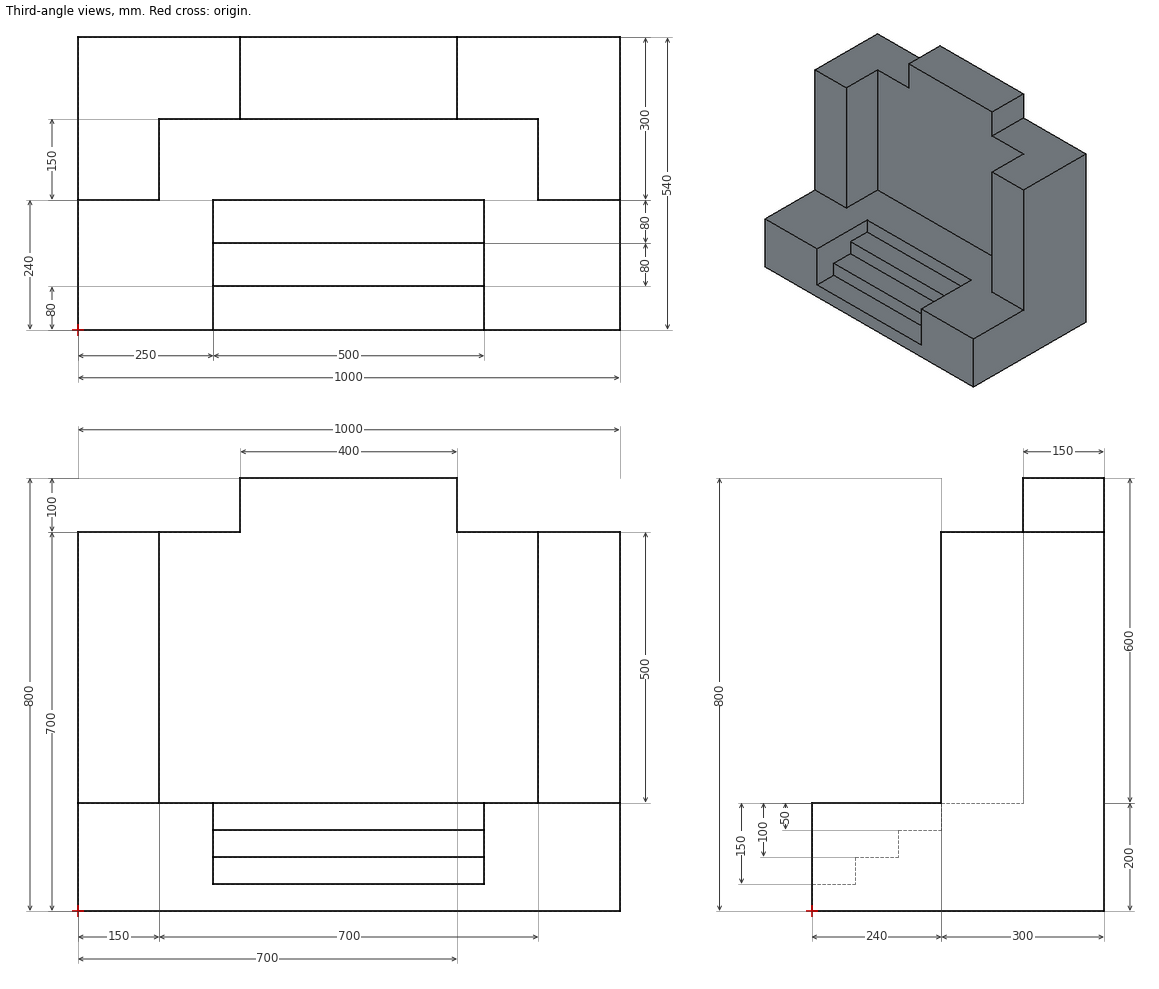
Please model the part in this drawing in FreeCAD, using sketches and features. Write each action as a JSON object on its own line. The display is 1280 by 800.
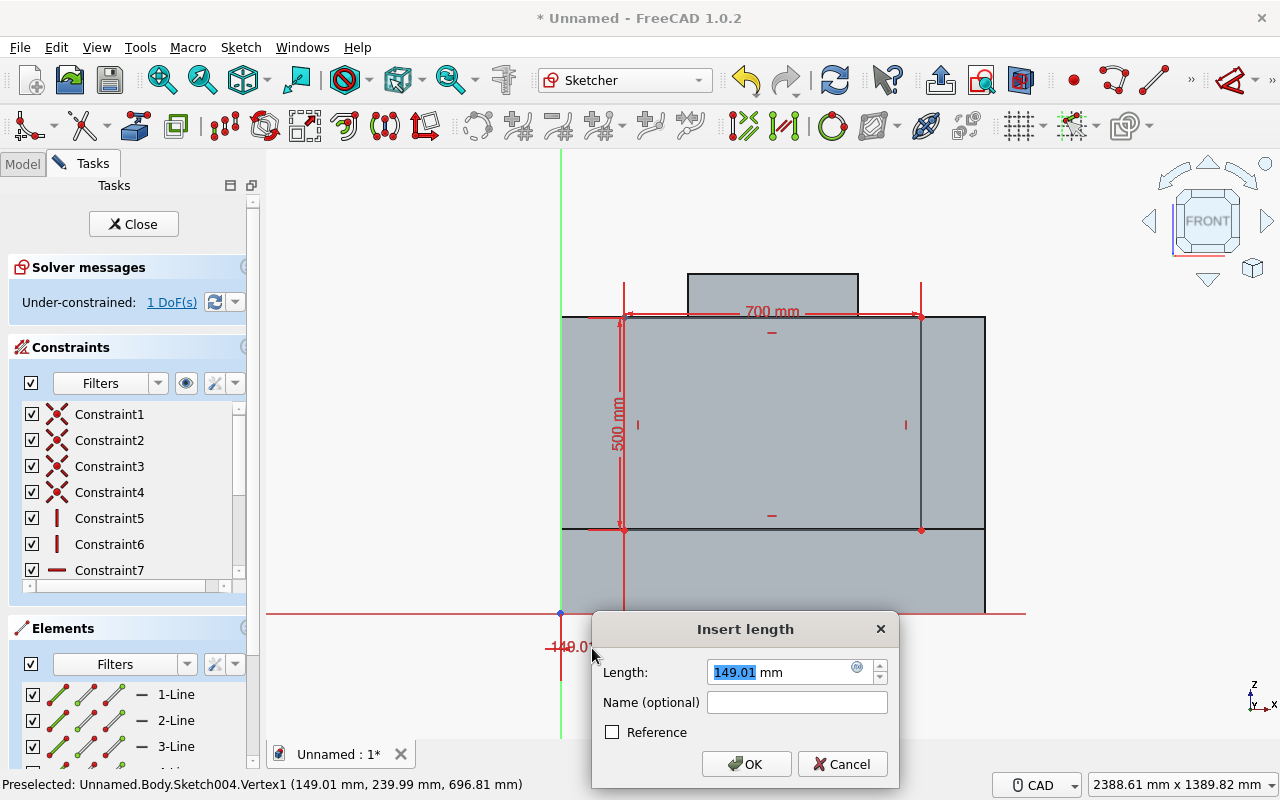
{"action": "type", "text": "150"}
{"action": "key", "text": "Return"}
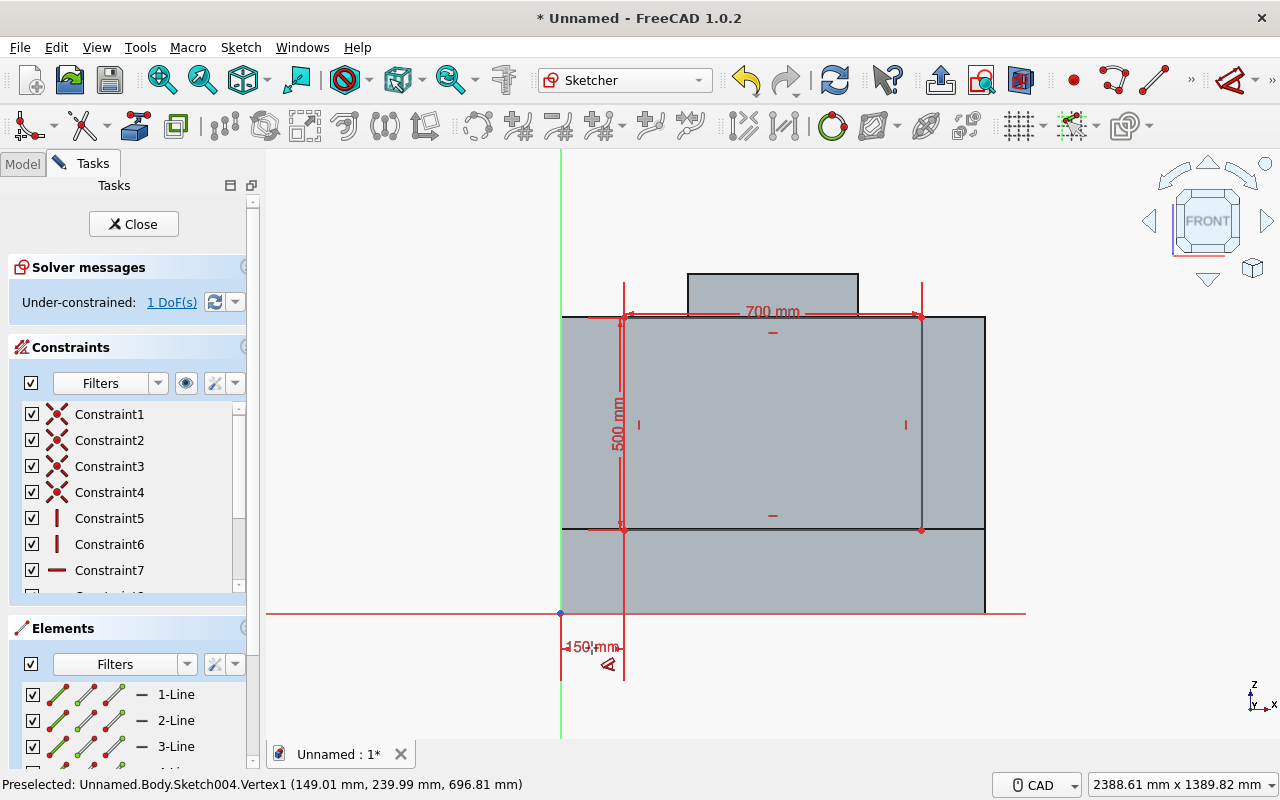
{"action": "left_click", "coordinate": [624, 318]}
{"action": "left_click", "coordinate": [527, 466]}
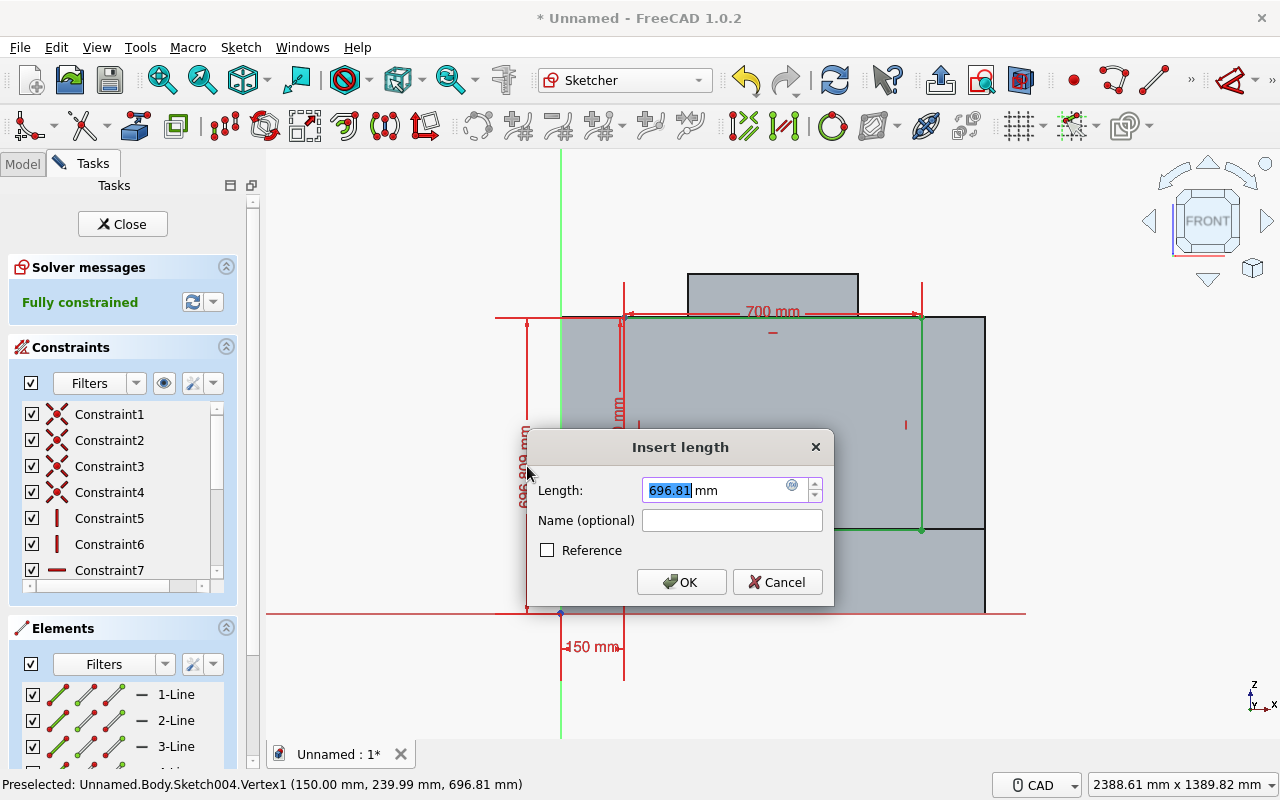
{"action": "type", "text": "700"}
{"action": "key", "text": "Return"}
{"action": "key", "text": "Escape"}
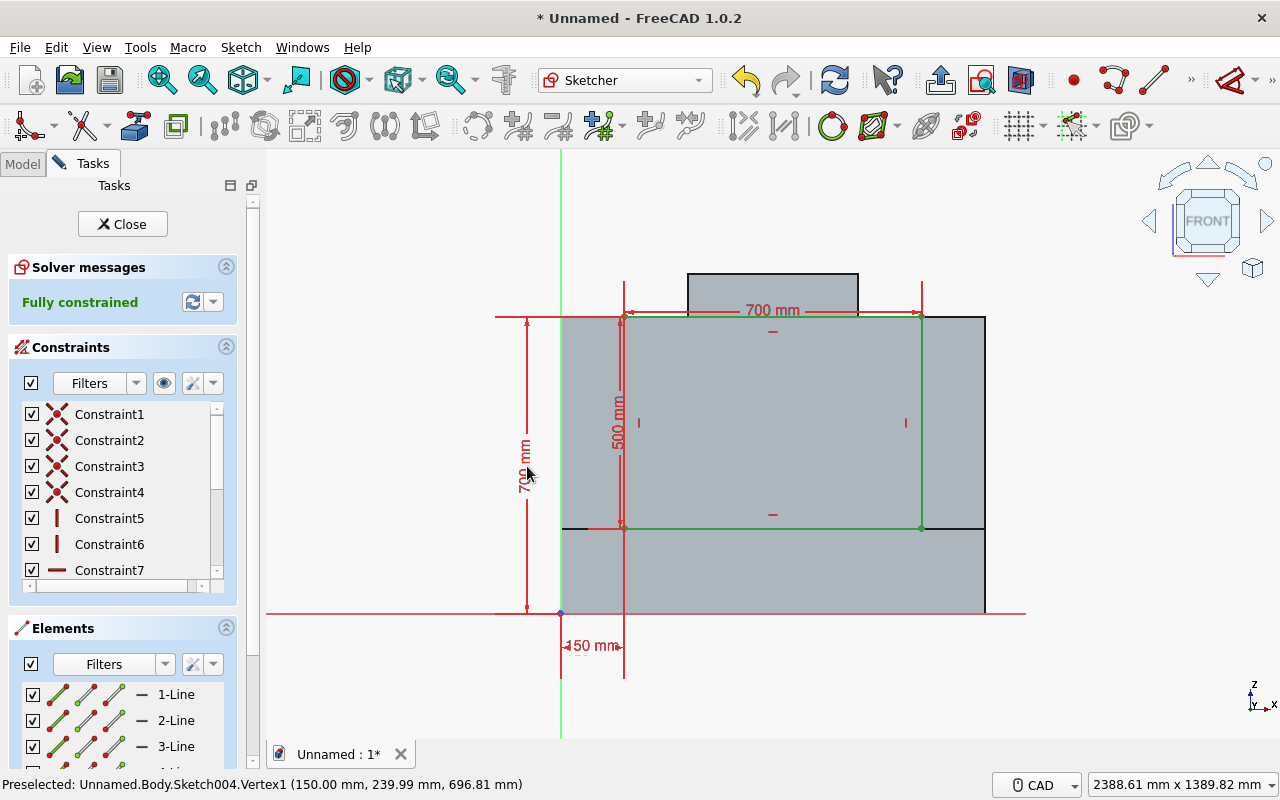
{"action": "left_click", "coordinate": [123, 224]}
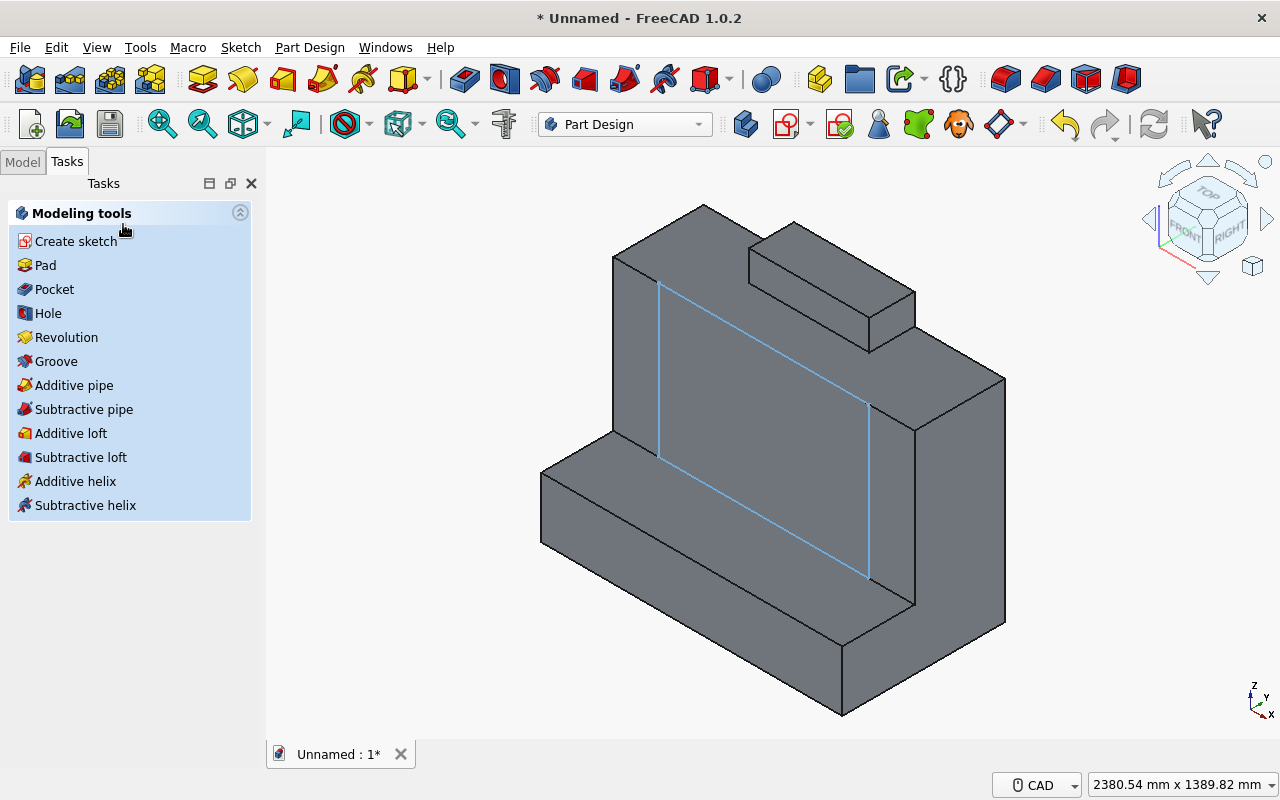
{"action": "left_click", "coordinate": [466, 80]}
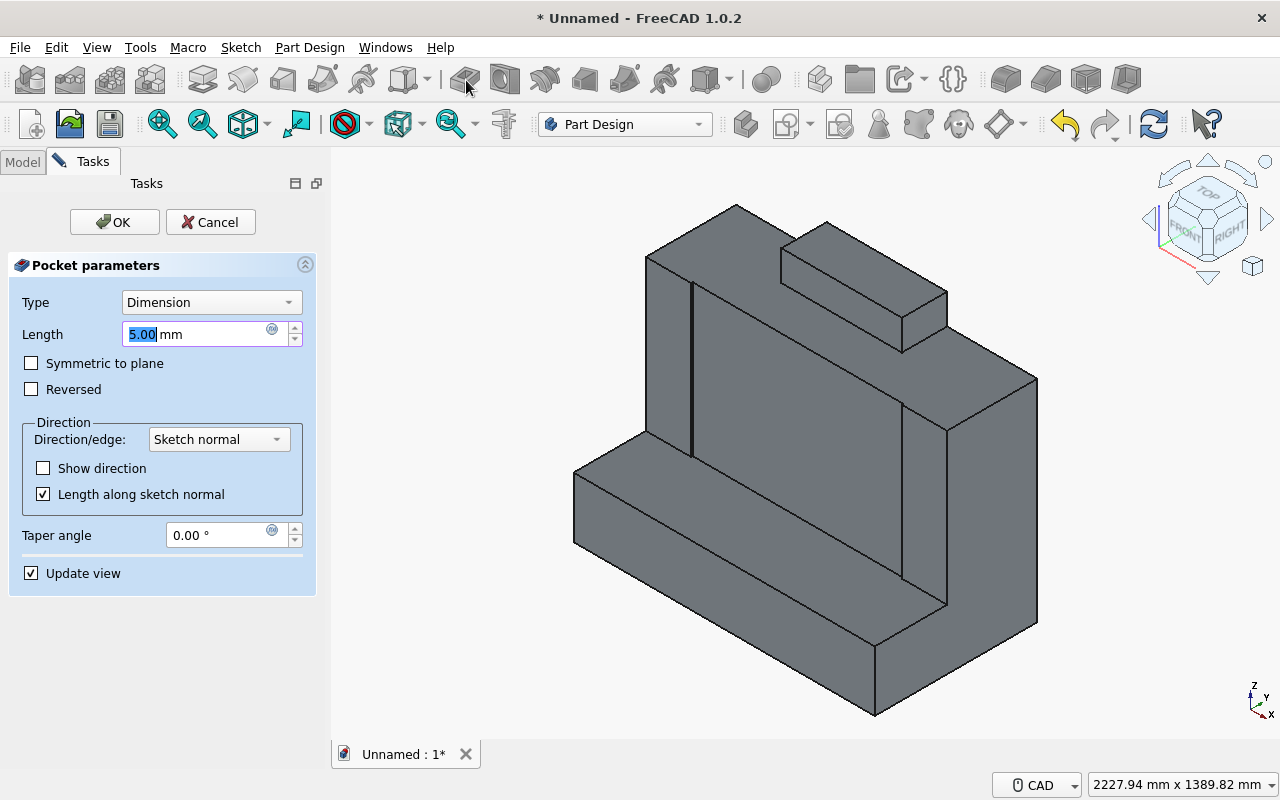
{"action": "type", "text": "150"}
{"action": "key", "text": "Tab"}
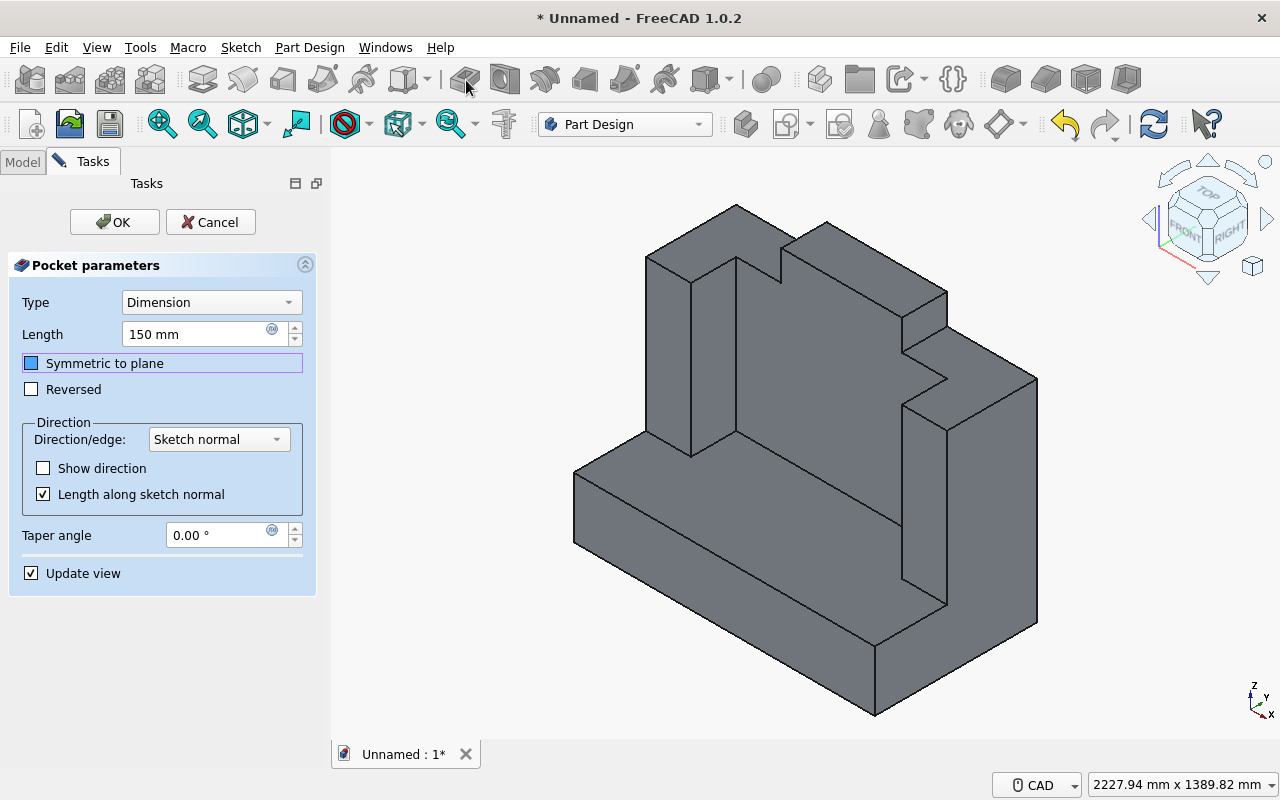
{"action": "left_click", "coordinate": [115, 222]}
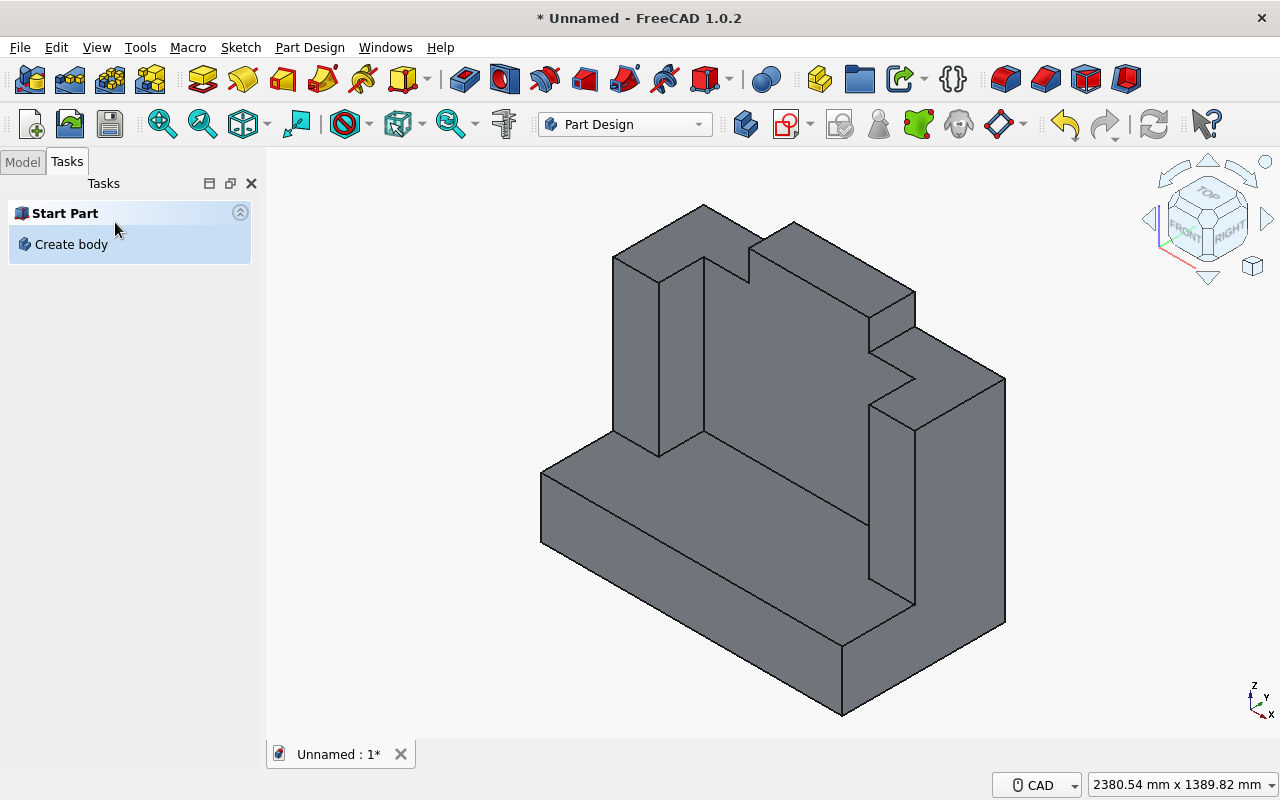
{"action": "left_click", "coordinate": [793, 549]}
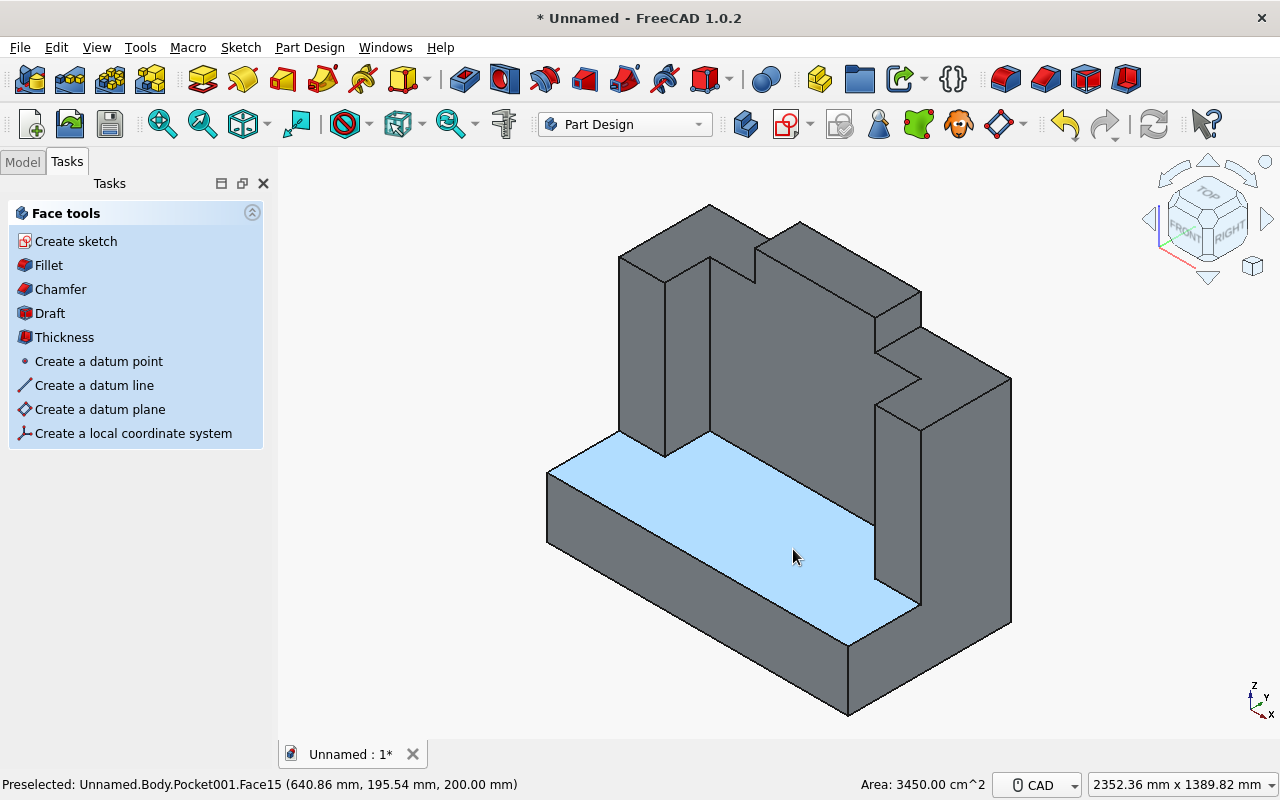
{"action": "left_click", "coordinate": [786, 124]}